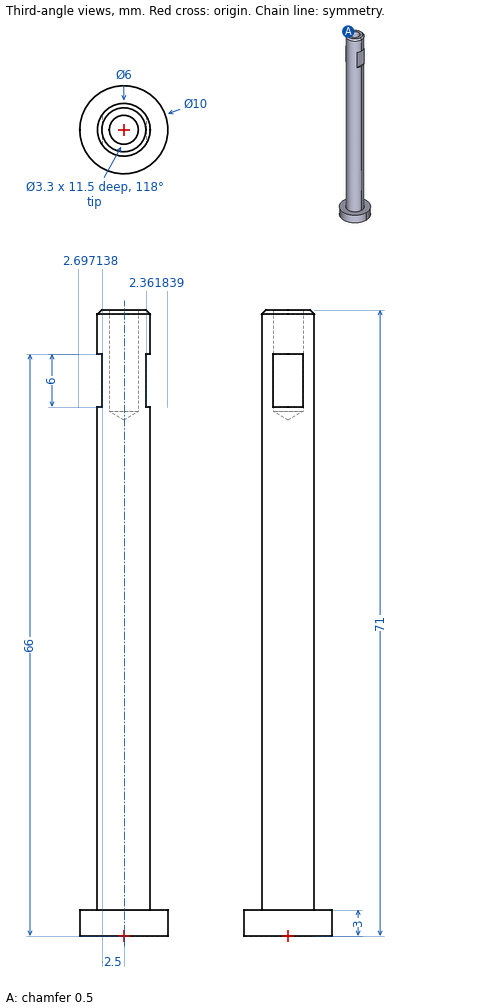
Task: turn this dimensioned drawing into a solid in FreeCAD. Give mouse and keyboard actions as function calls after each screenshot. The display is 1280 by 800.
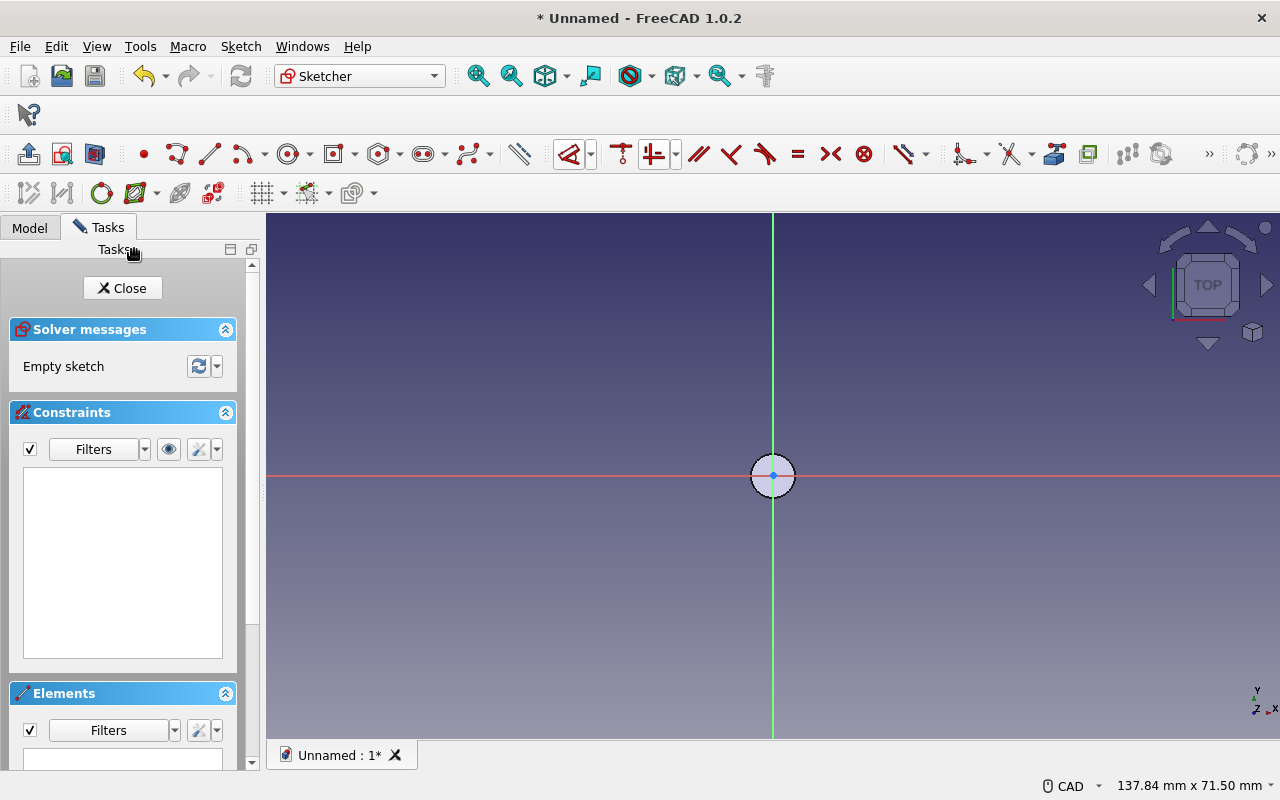
scroll(790, 476, up, 8)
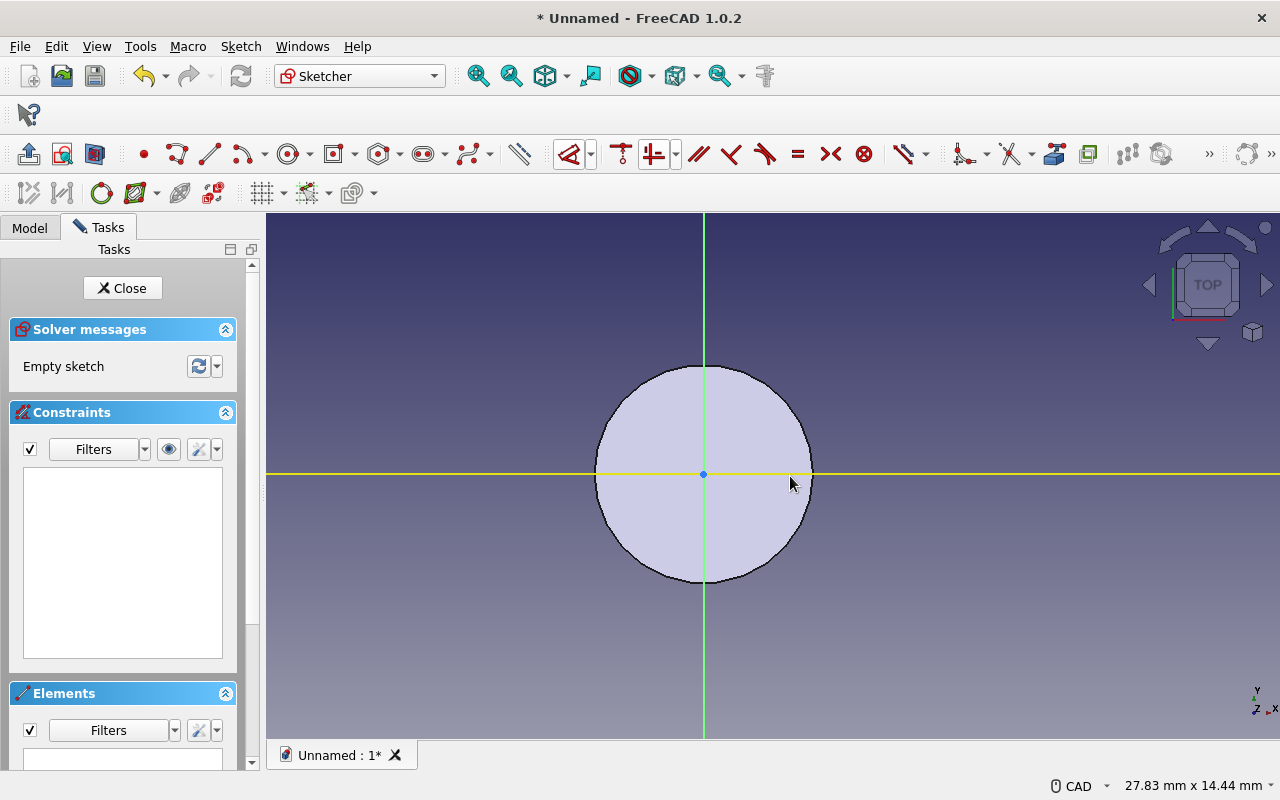
key(g)
key(c)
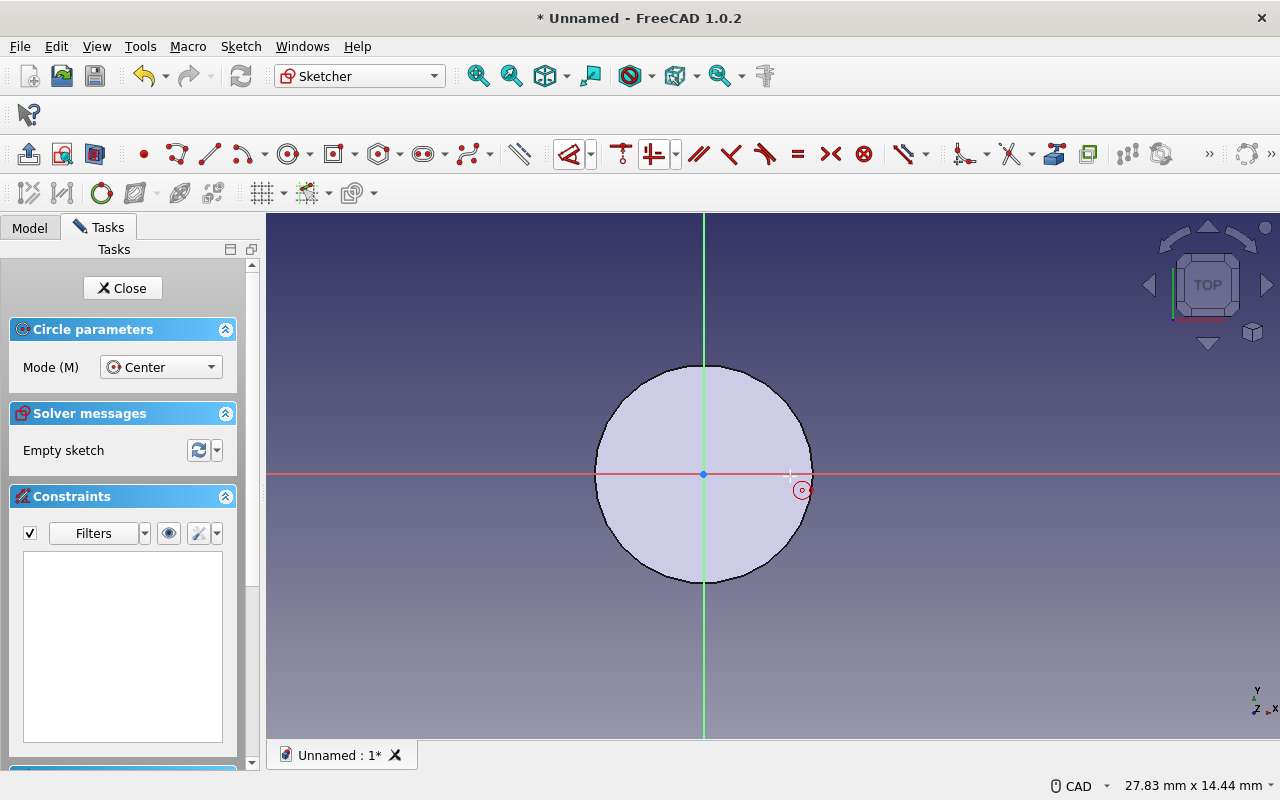
click(704, 474)
move(833, 345)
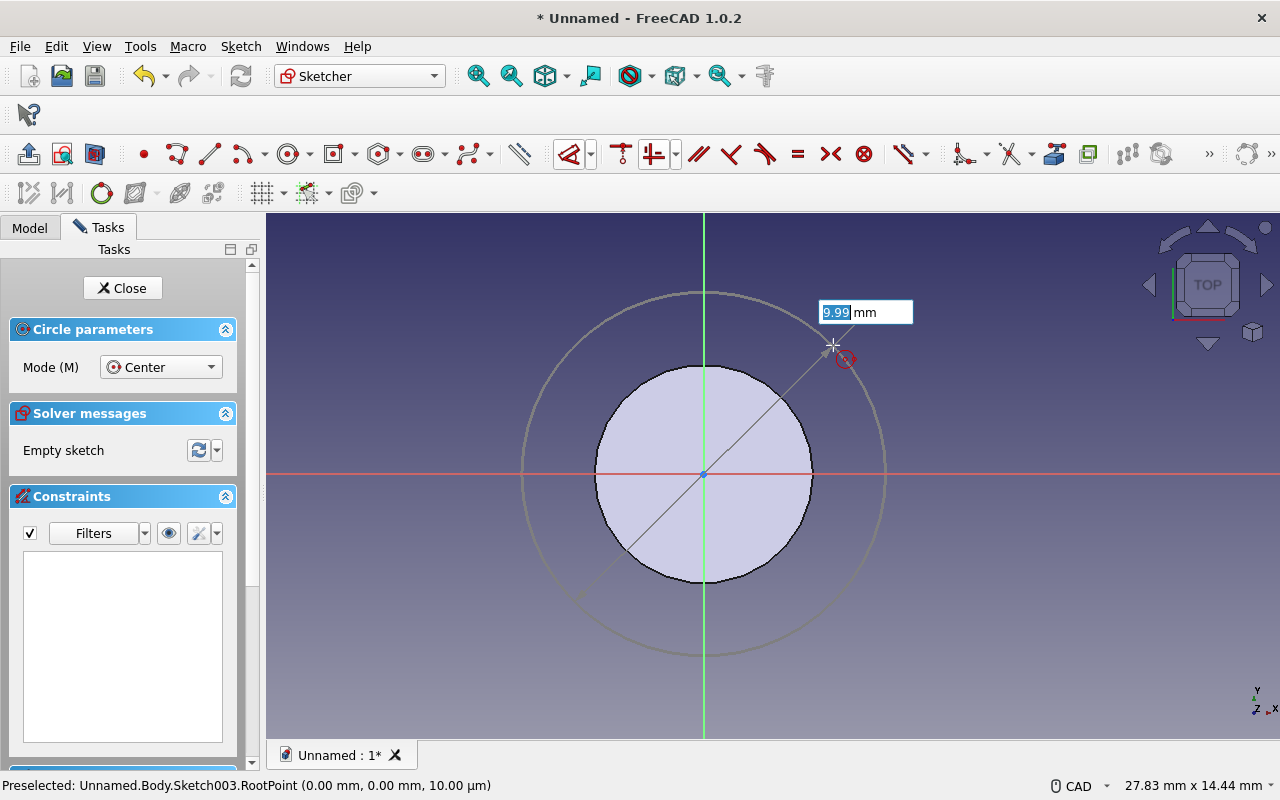
text(10)
key(Return)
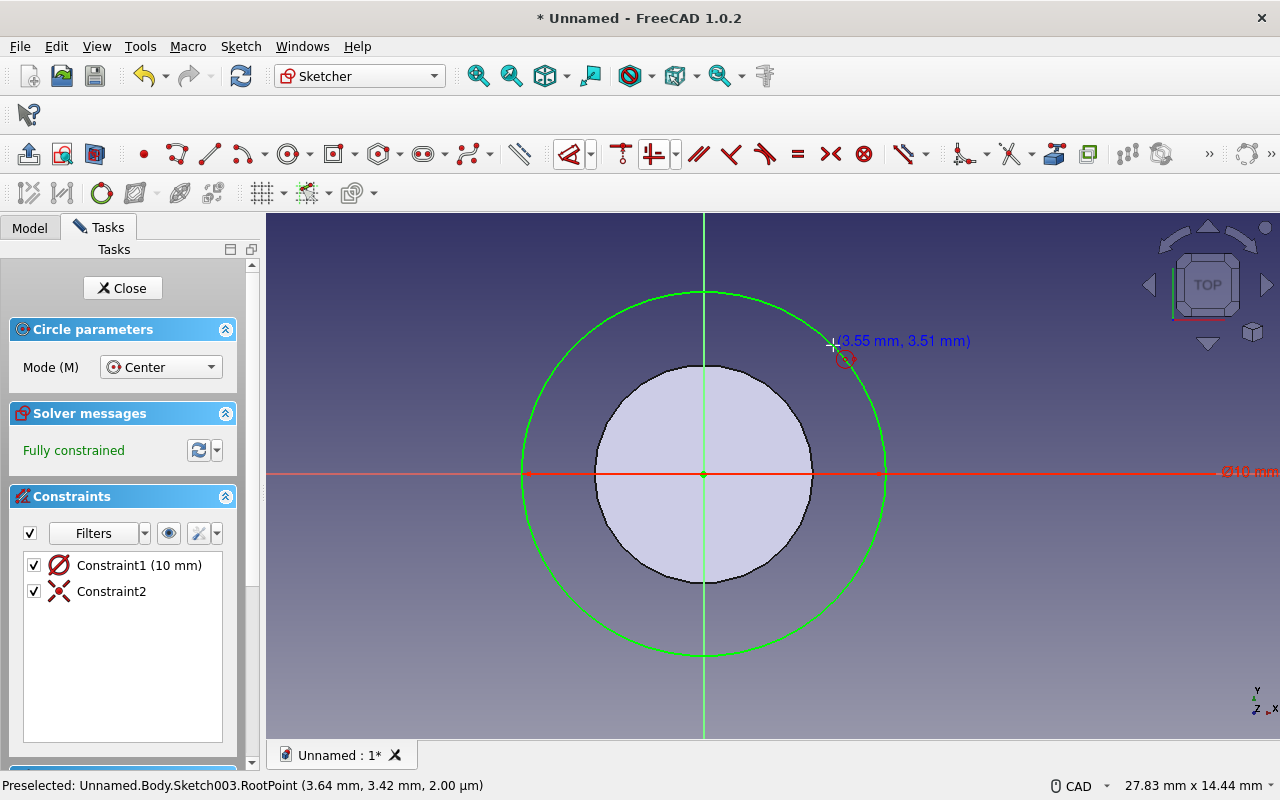
click(704, 474)
move(781, 397)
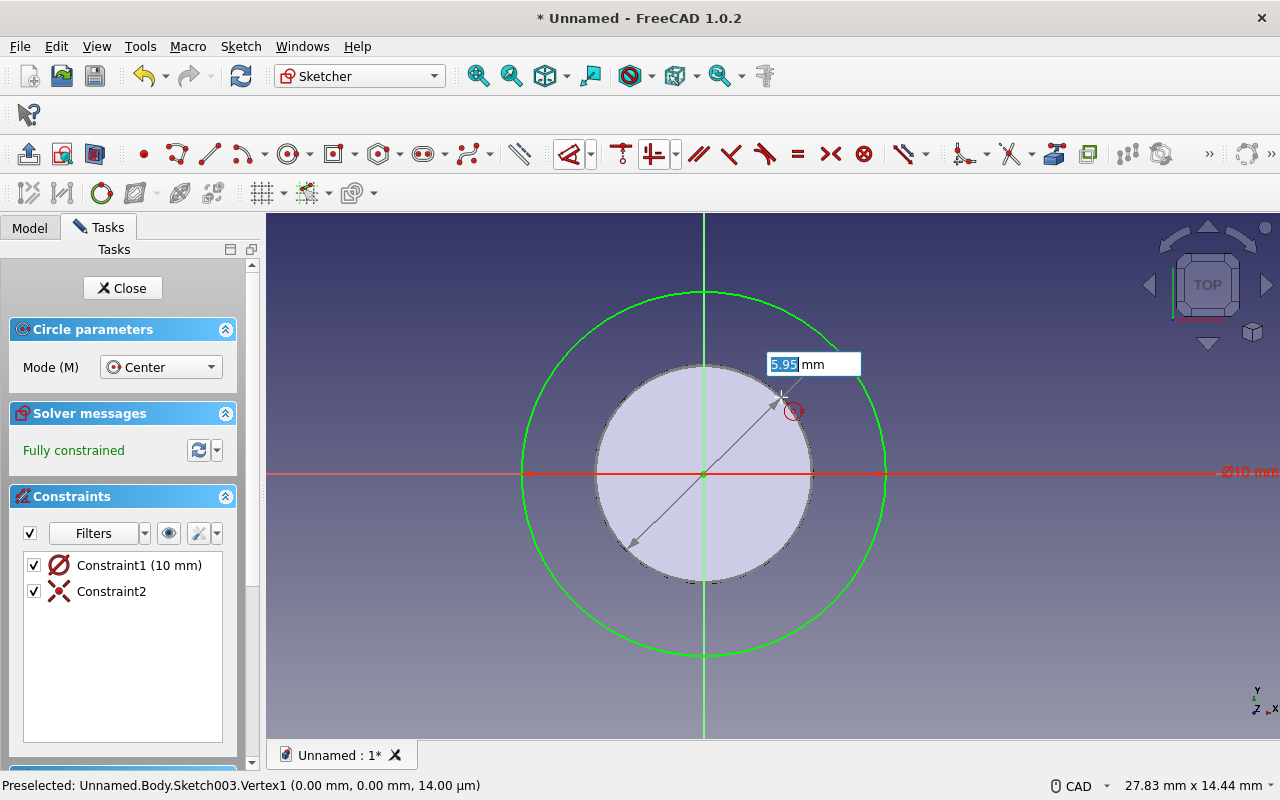
text(6)
key(Return)
key(Escape)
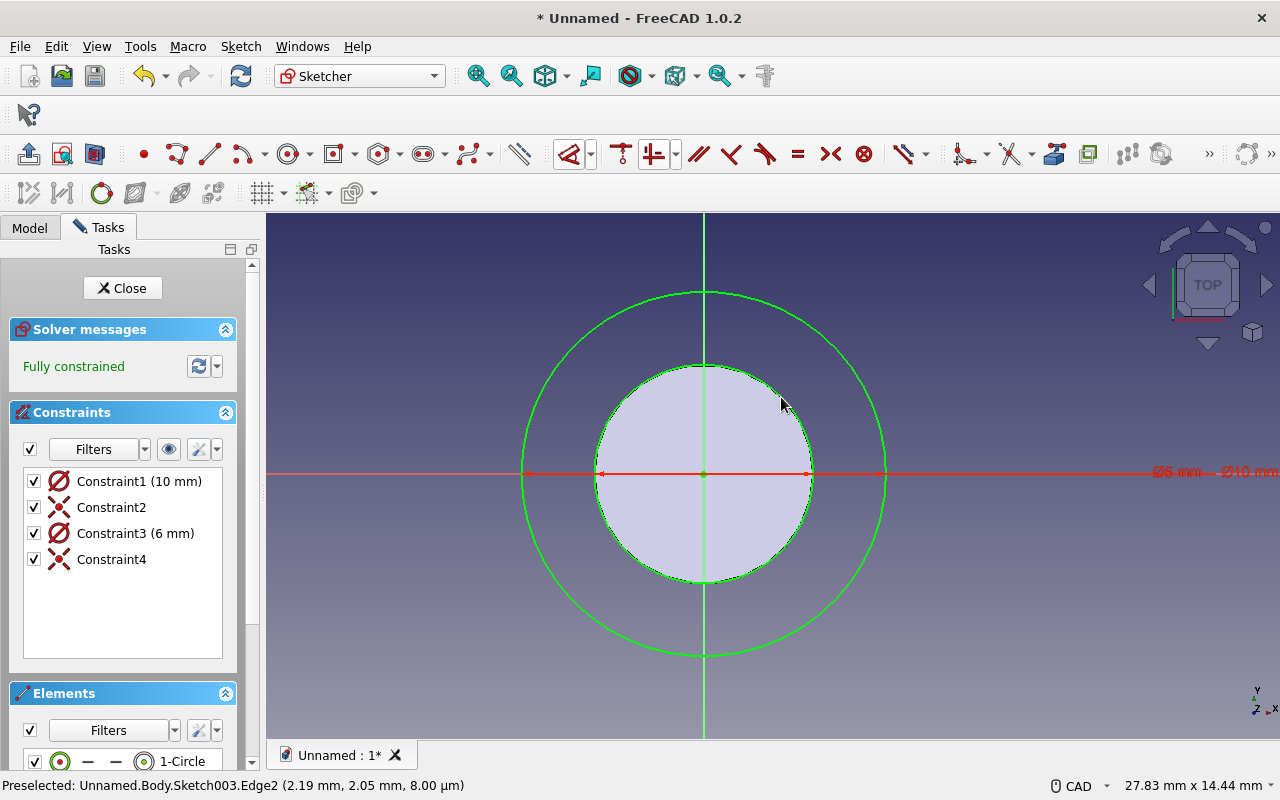
click(123, 288)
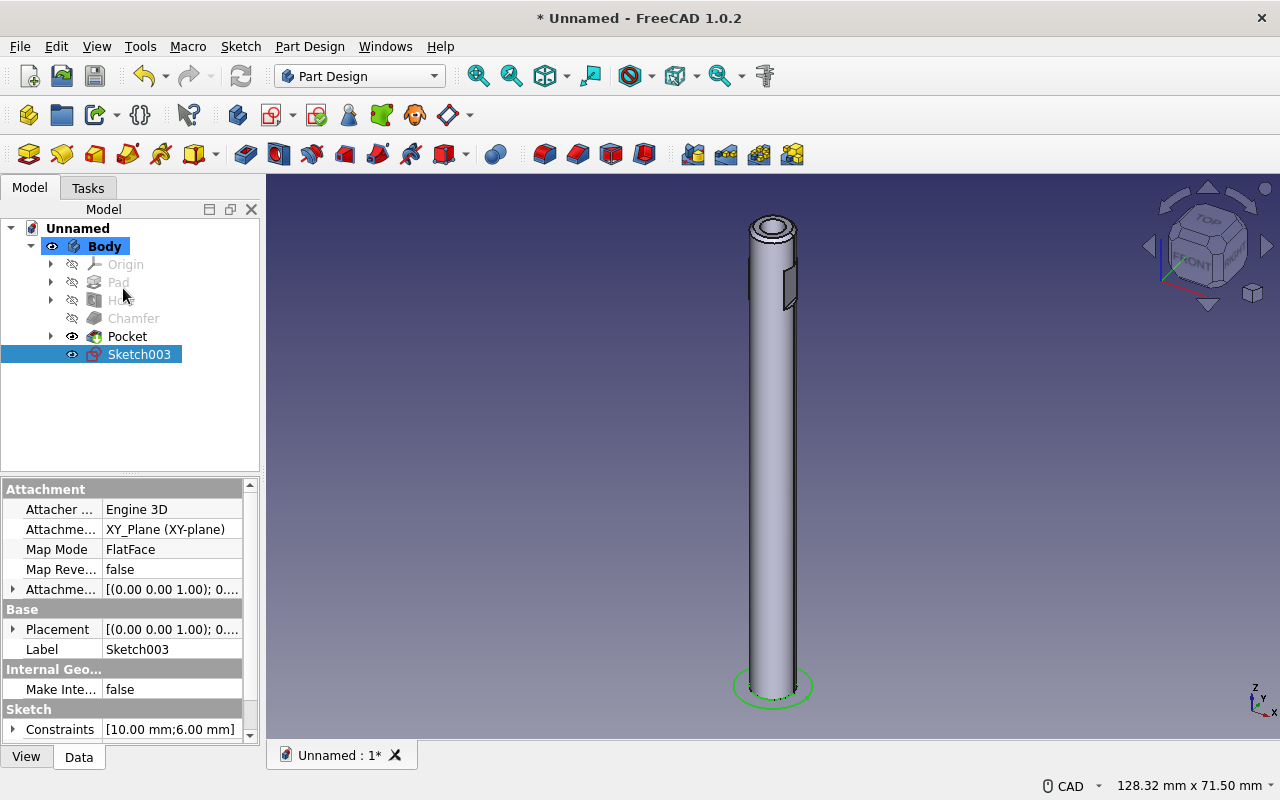
click(29, 154)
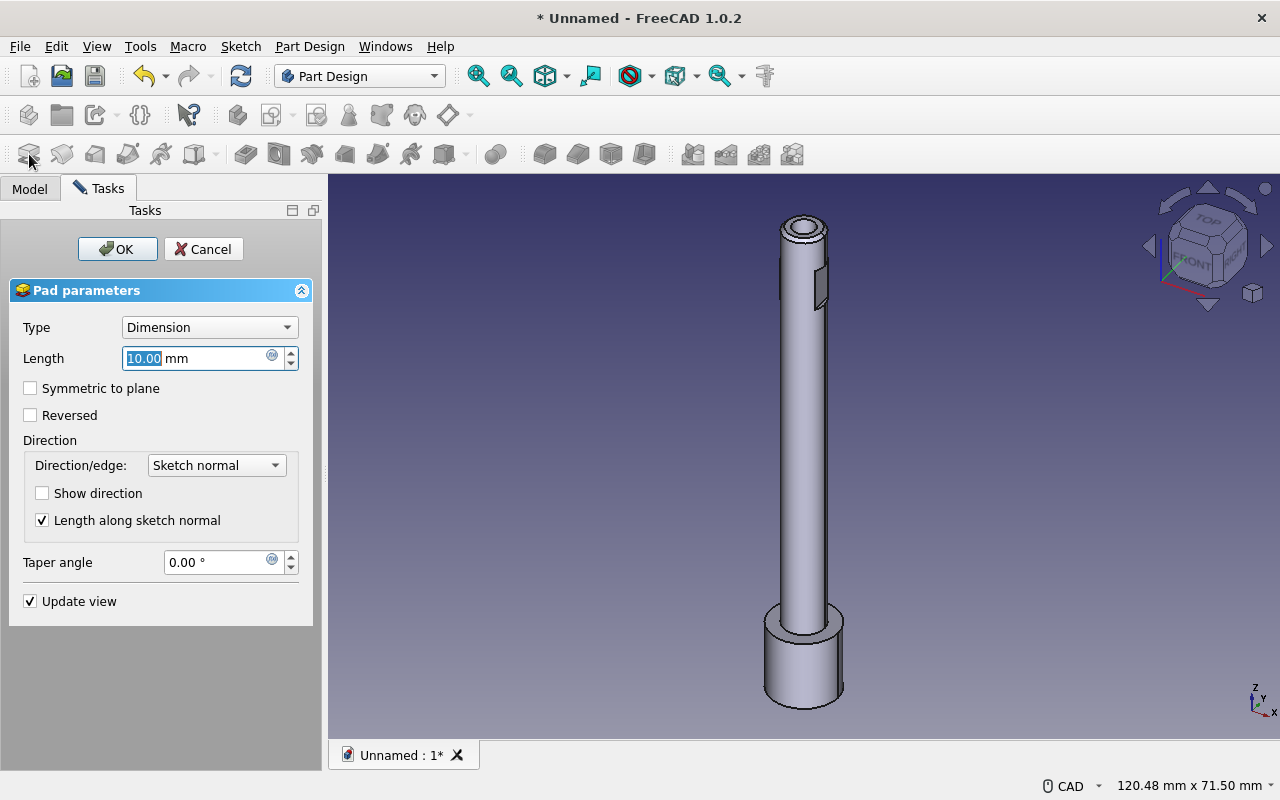
text(3)
key(Tab)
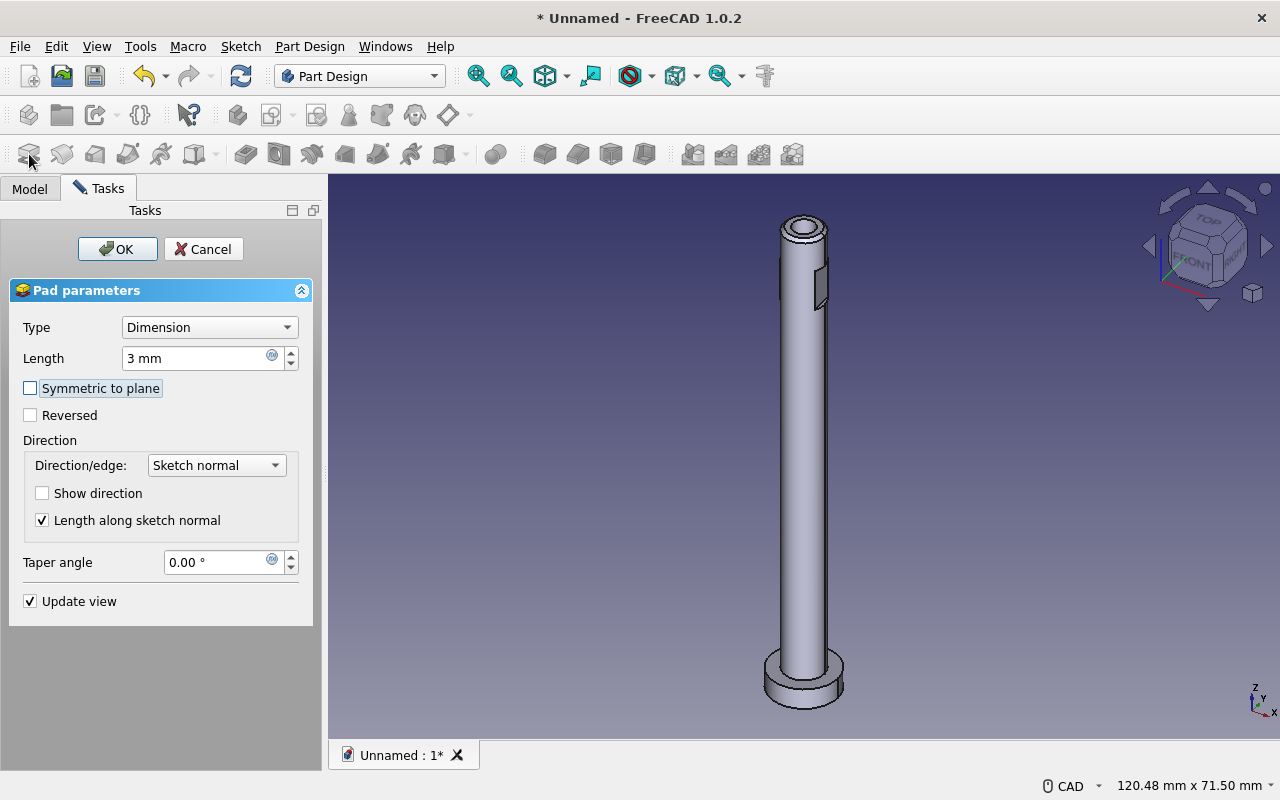
click(118, 249)